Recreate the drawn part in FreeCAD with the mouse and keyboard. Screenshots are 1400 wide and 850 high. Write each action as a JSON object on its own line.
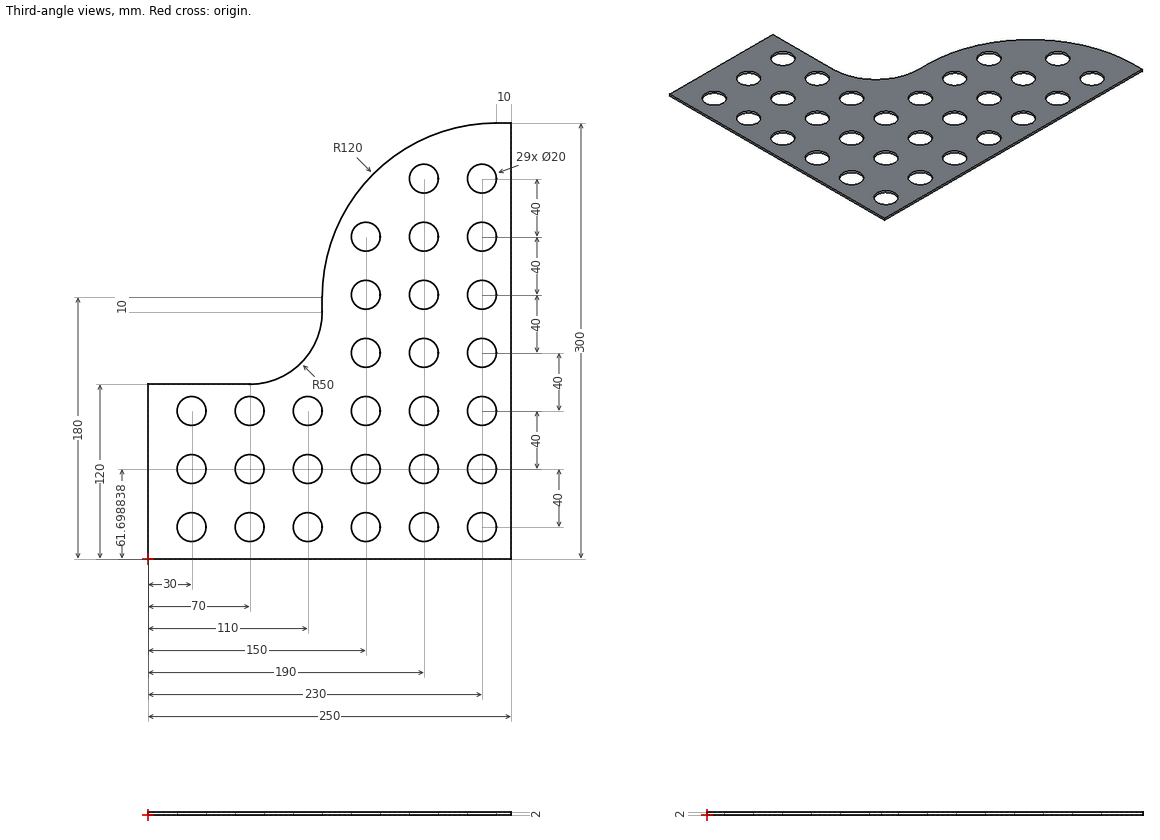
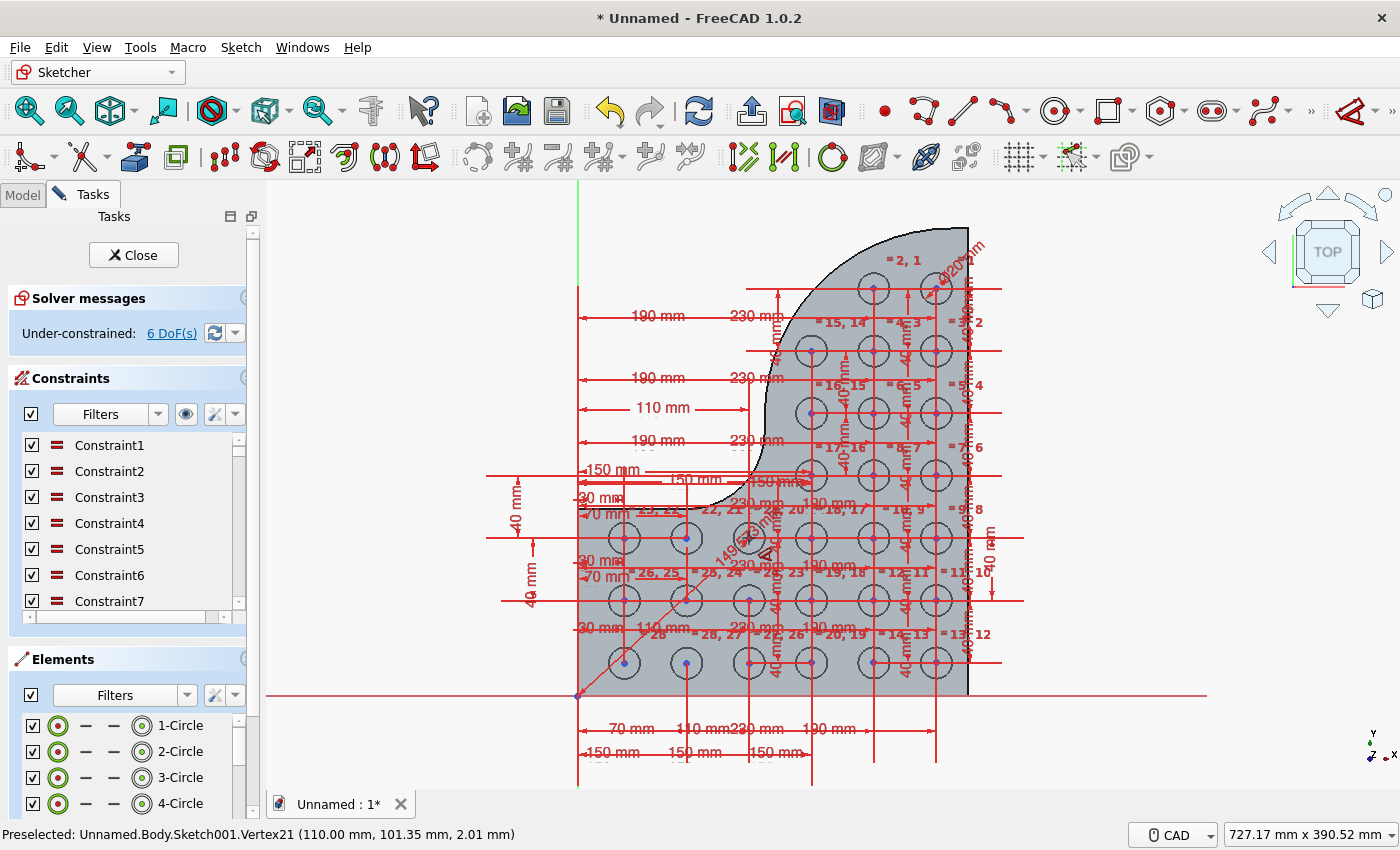
{"action": "left_click", "coordinate": [749, 601]}
{"action": "left_click", "coordinate": [715, 570]}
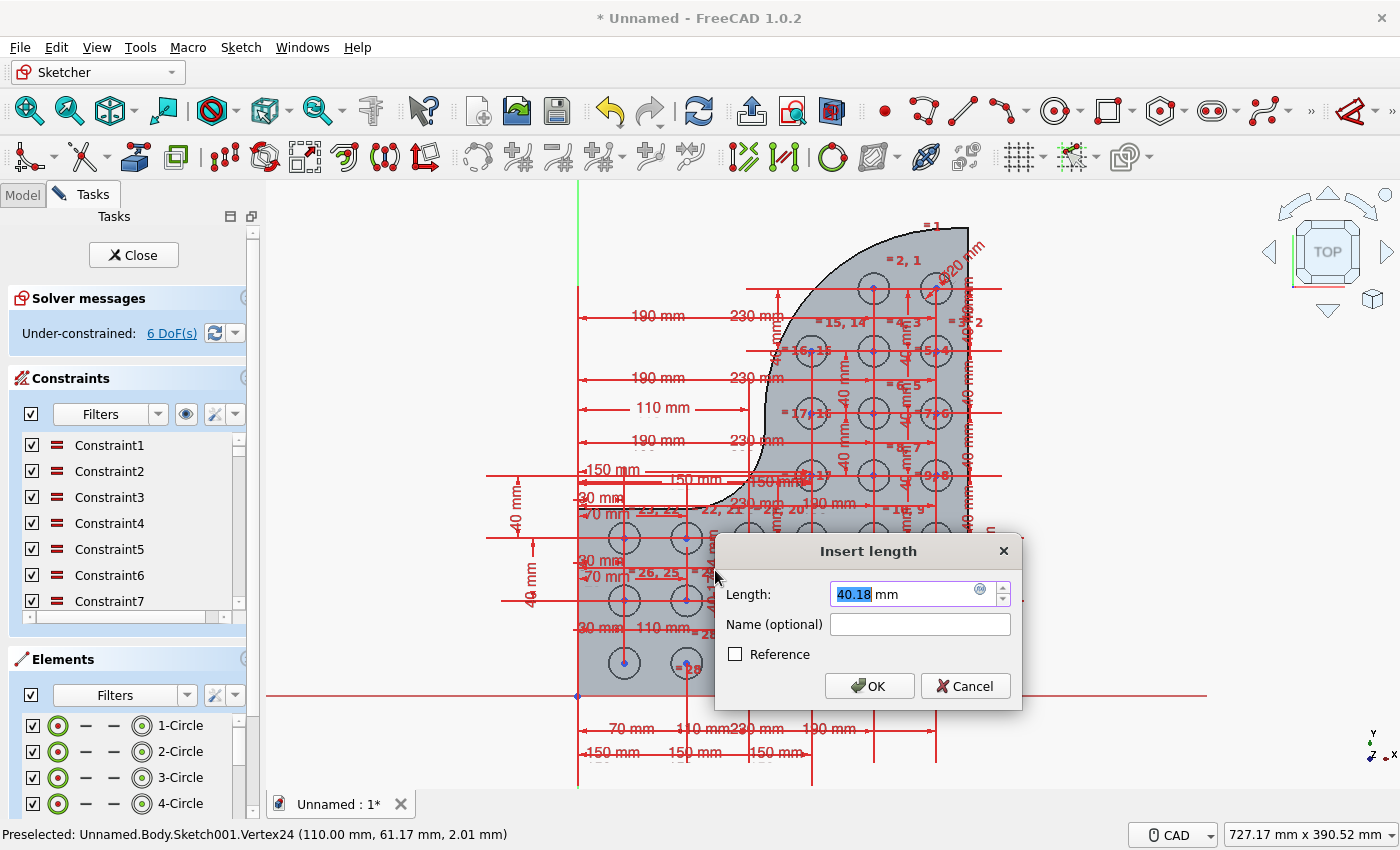
{"action": "type", "text": "40"}
{"action": "key", "text": "Return"}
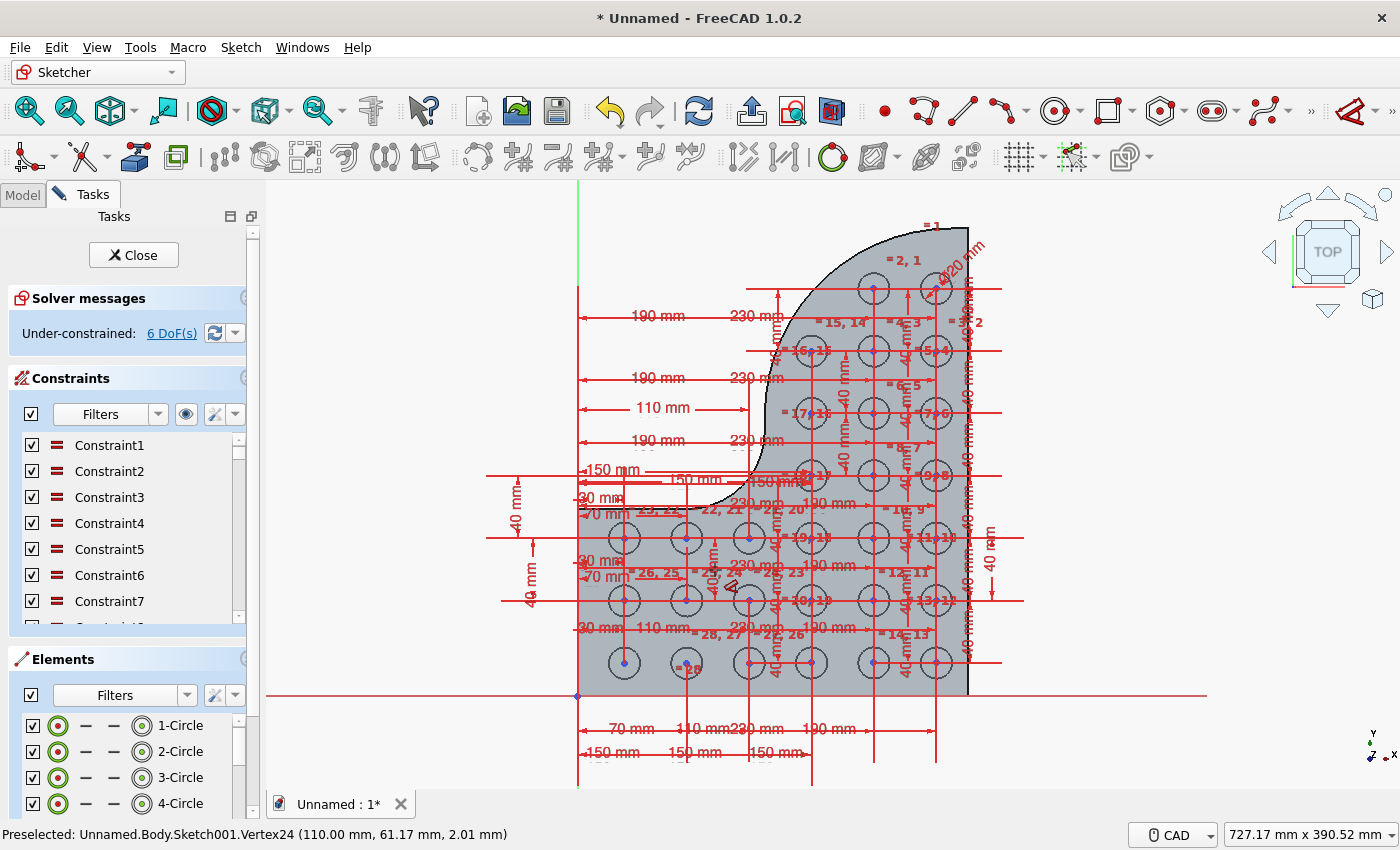
{"action": "left_click", "coordinate": [687, 538]}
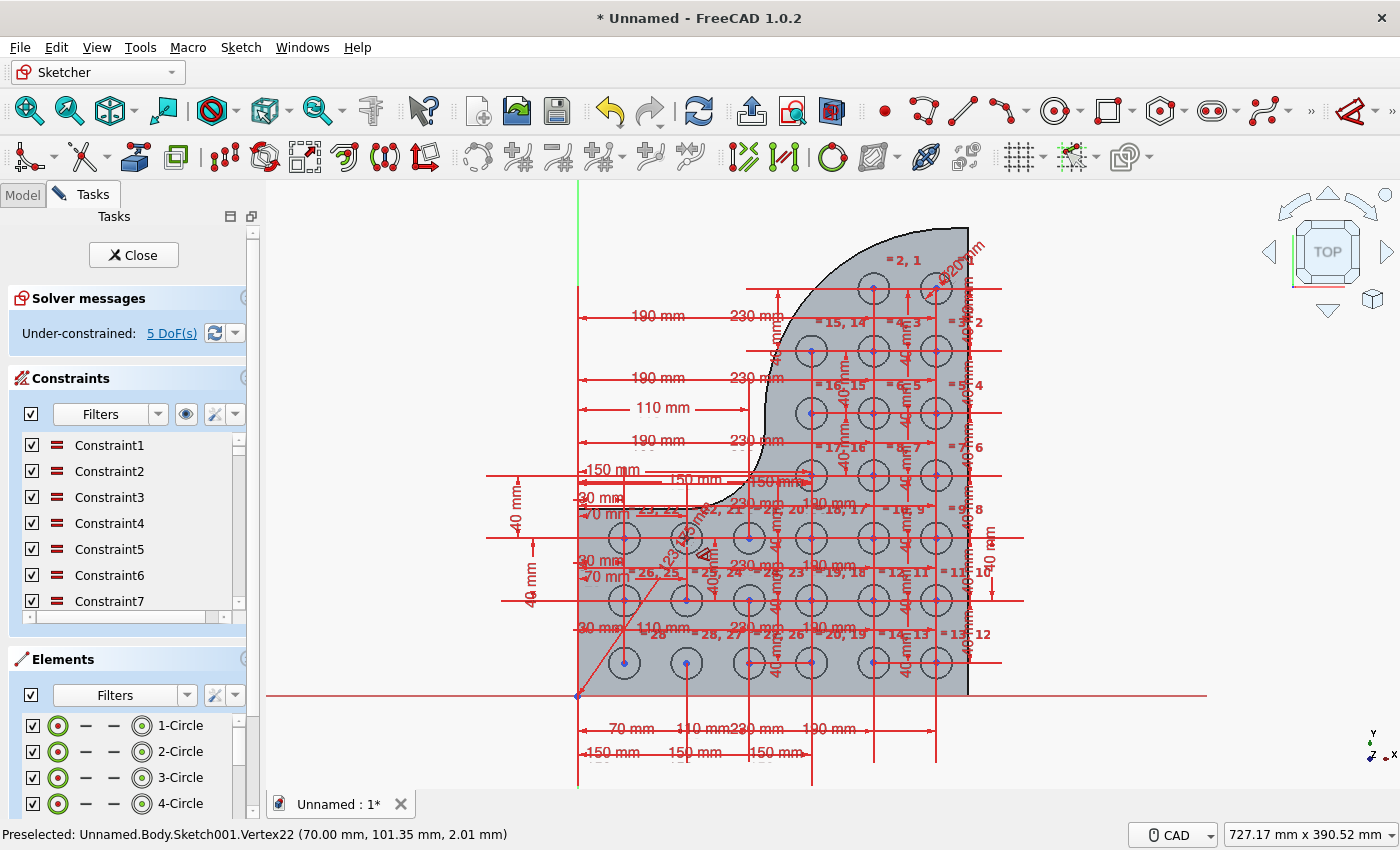
{"action": "left_click", "coordinate": [687, 601]}
{"action": "left_click", "coordinate": [507, 555]}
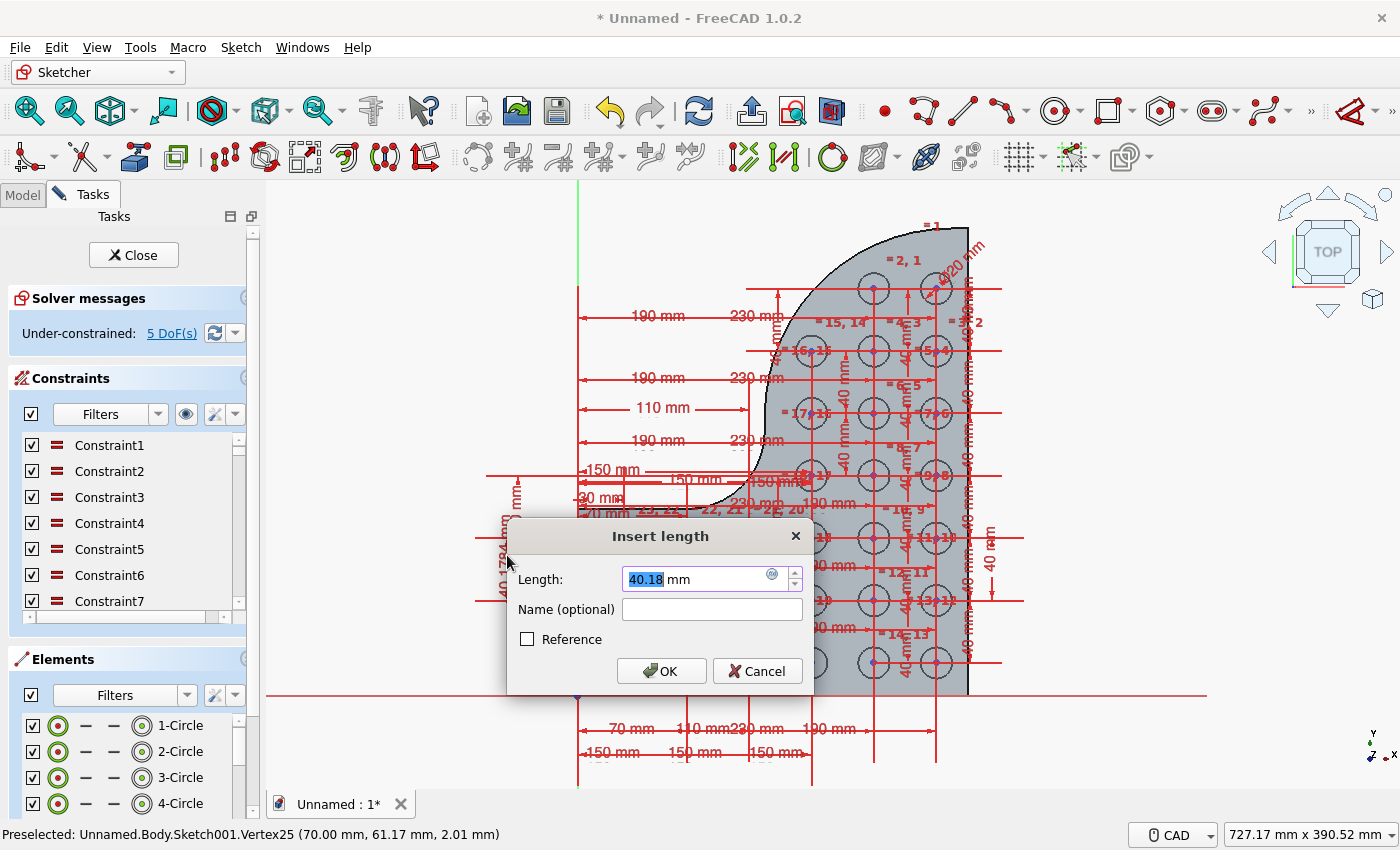
{"action": "type", "text": "40"}
{"action": "key", "text": "Return"}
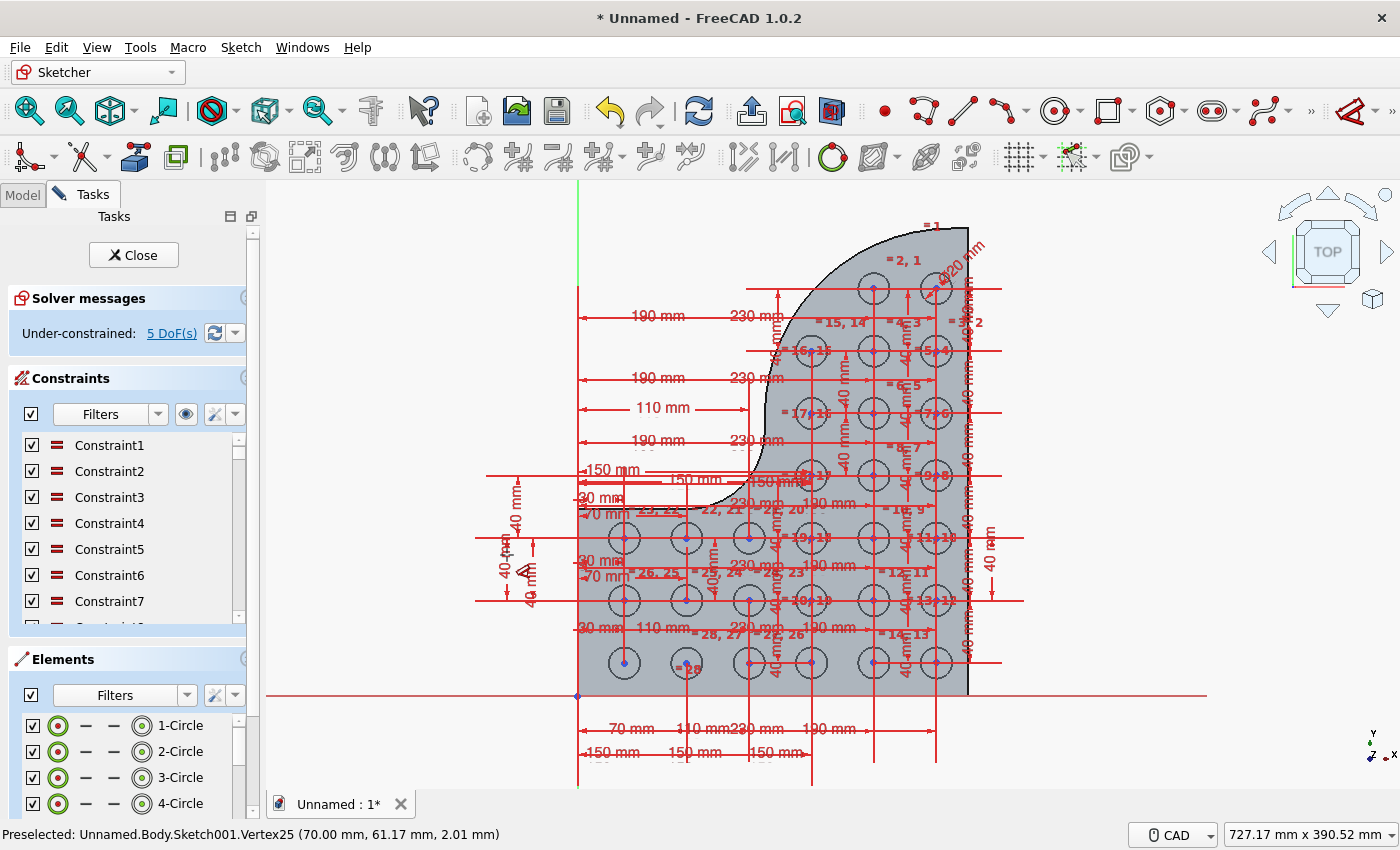
{"action": "left_click", "coordinate": [624, 538]}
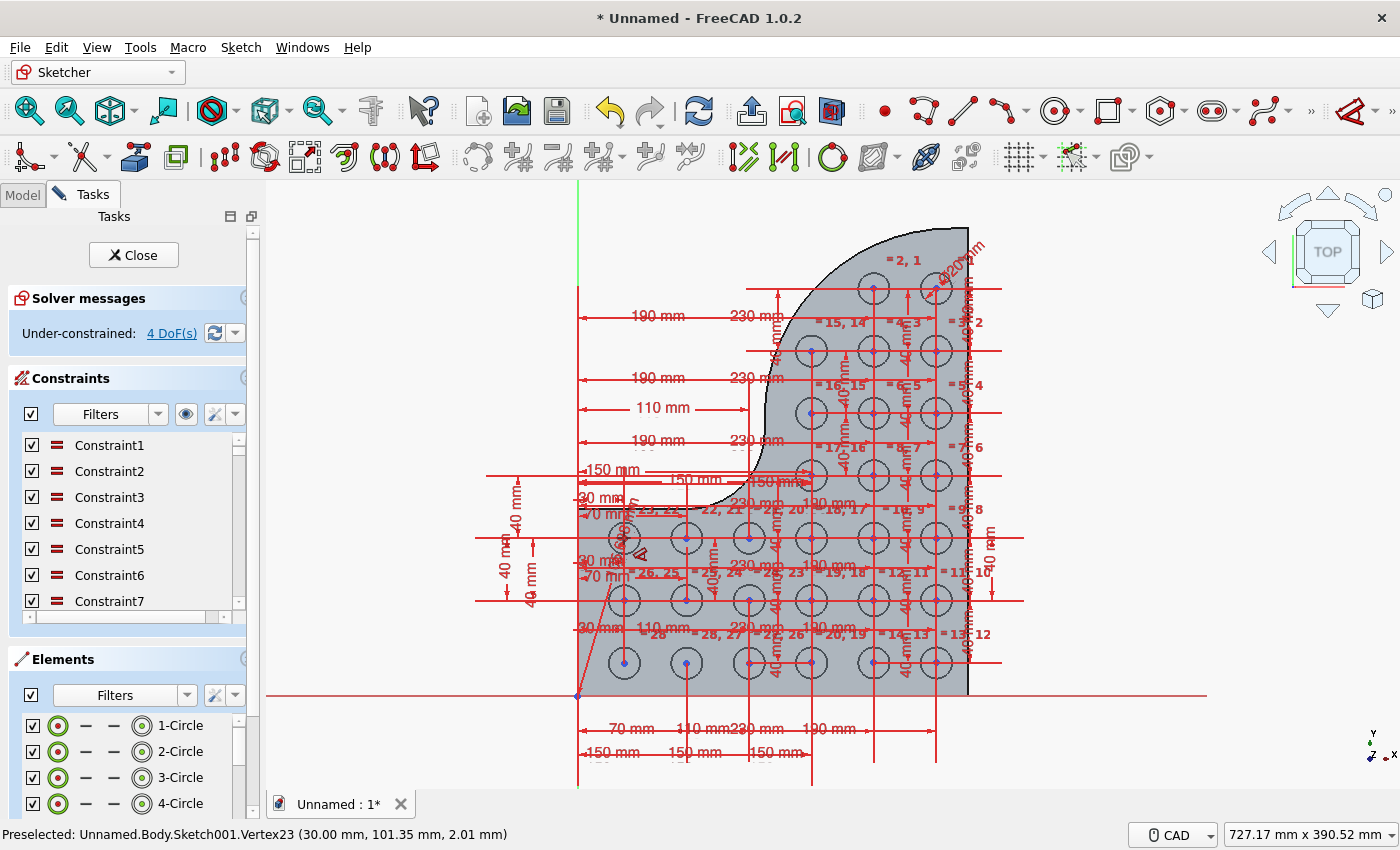
{"action": "left_click", "coordinate": [624, 601]}
{"action": "left_click", "coordinate": [444, 584]}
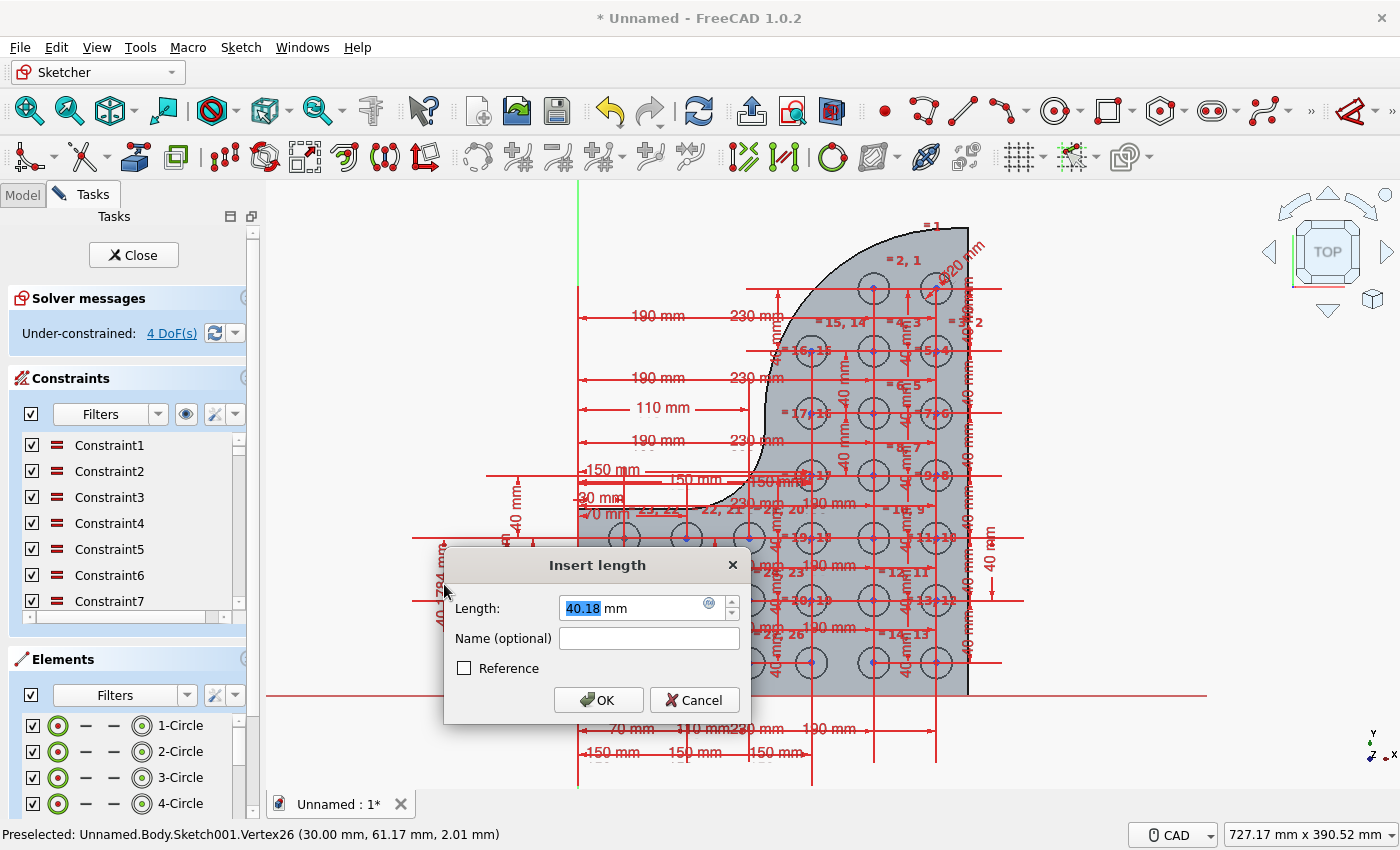
{"action": "type", "text": "40"}
{"action": "key", "text": "Return"}